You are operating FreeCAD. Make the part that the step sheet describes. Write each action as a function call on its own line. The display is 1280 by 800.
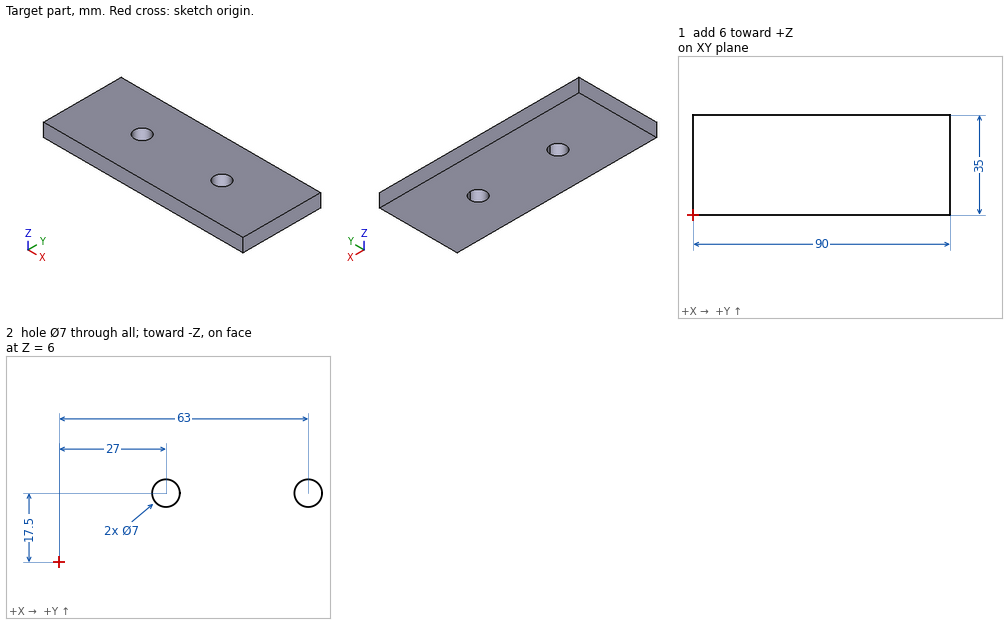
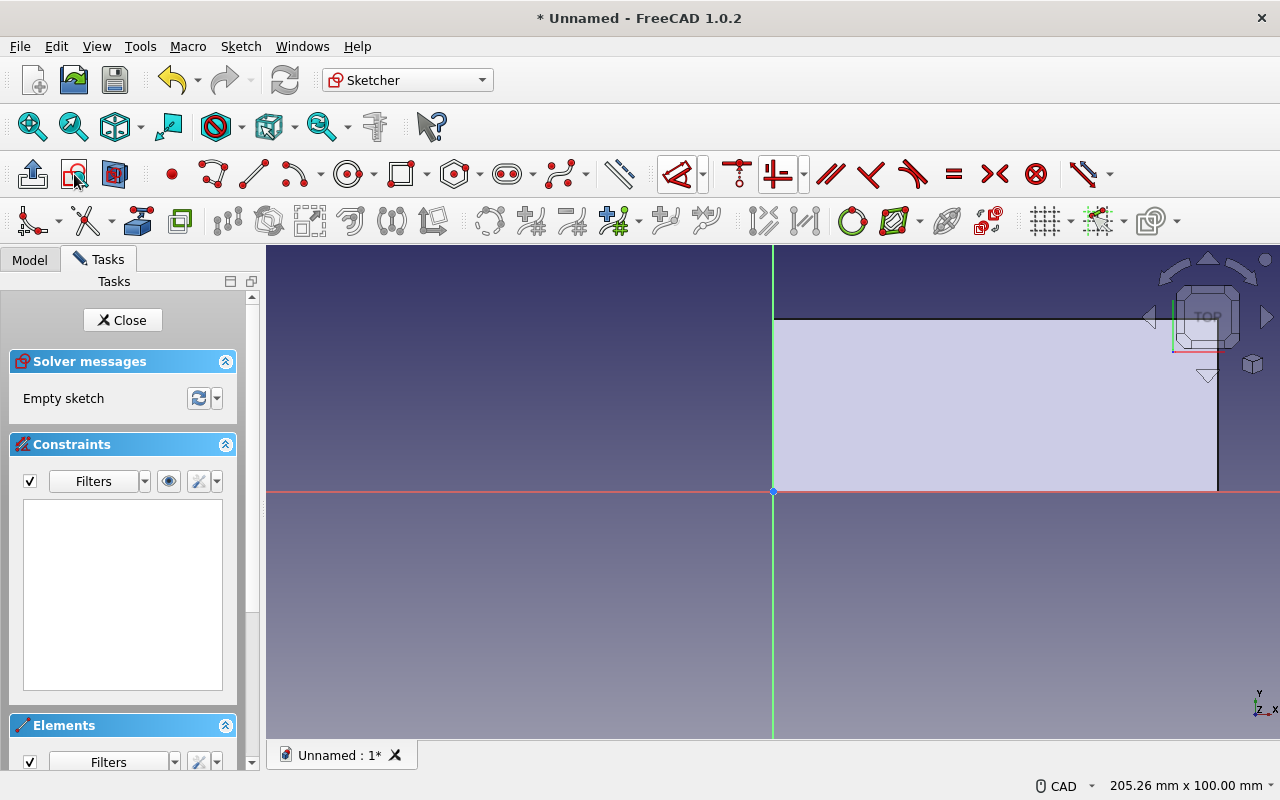
scroll(704, 492, down, 5)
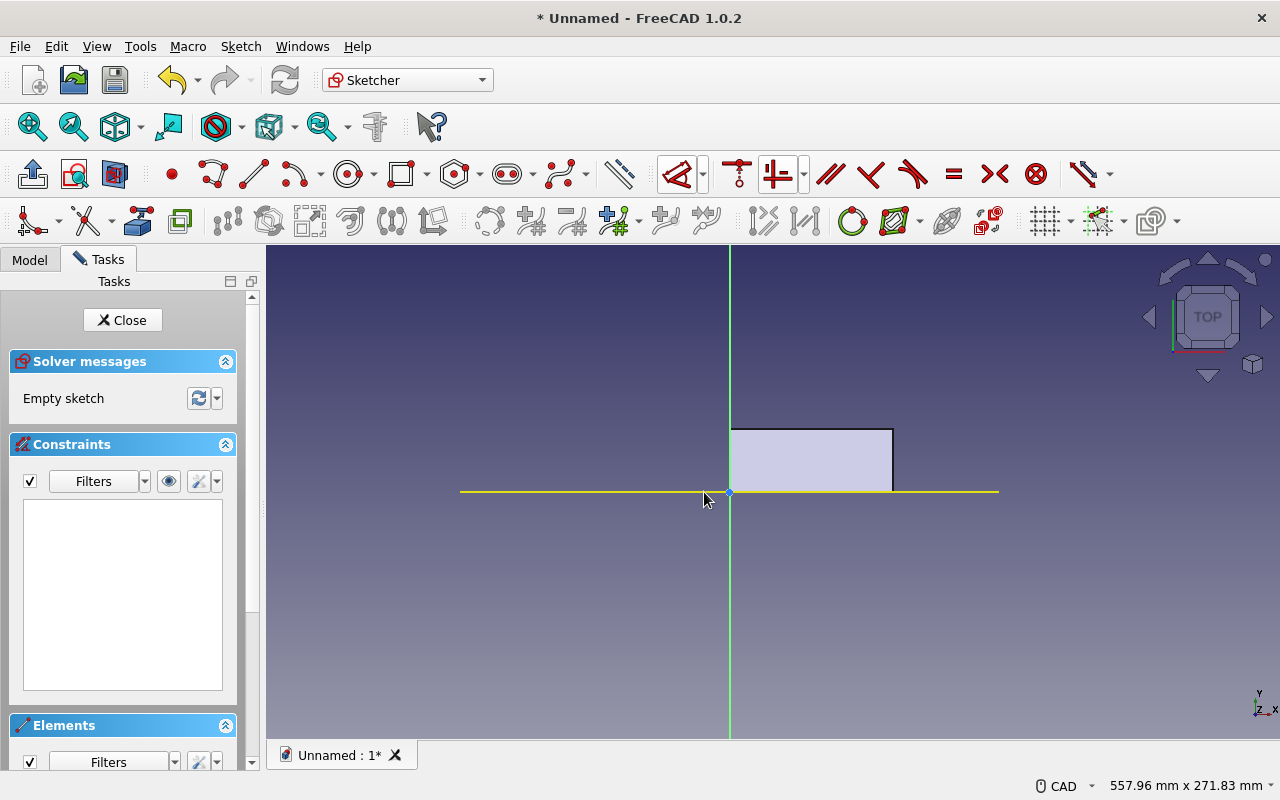
scroll(812, 468, up, 8)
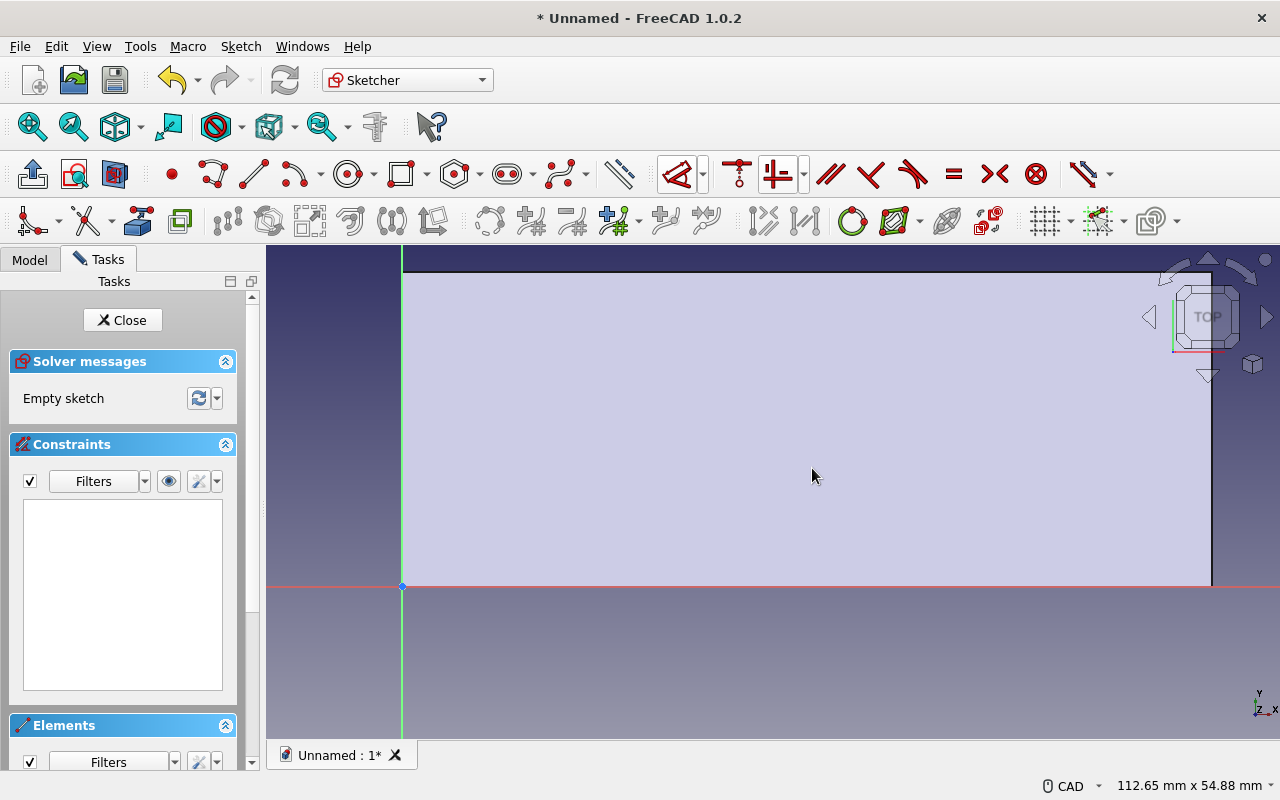
click(348, 174)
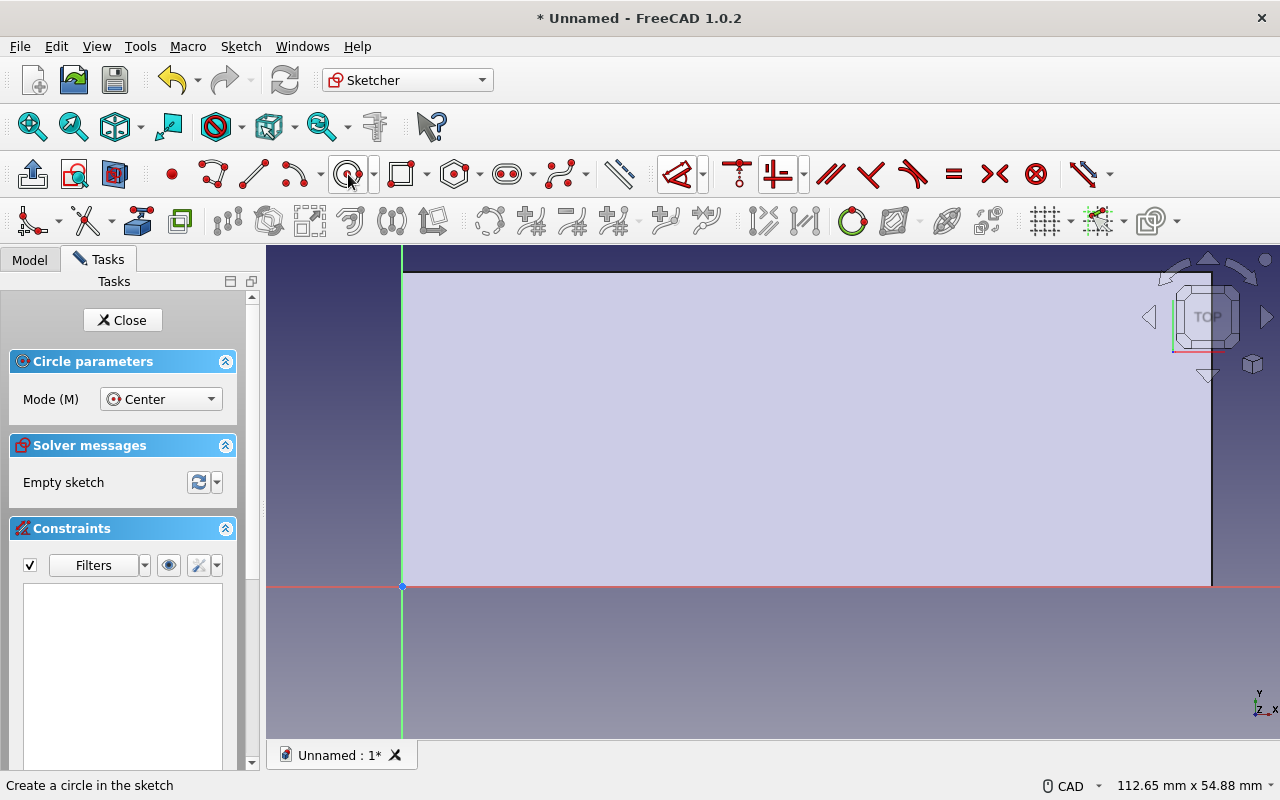
click(645, 429)
click(667, 407)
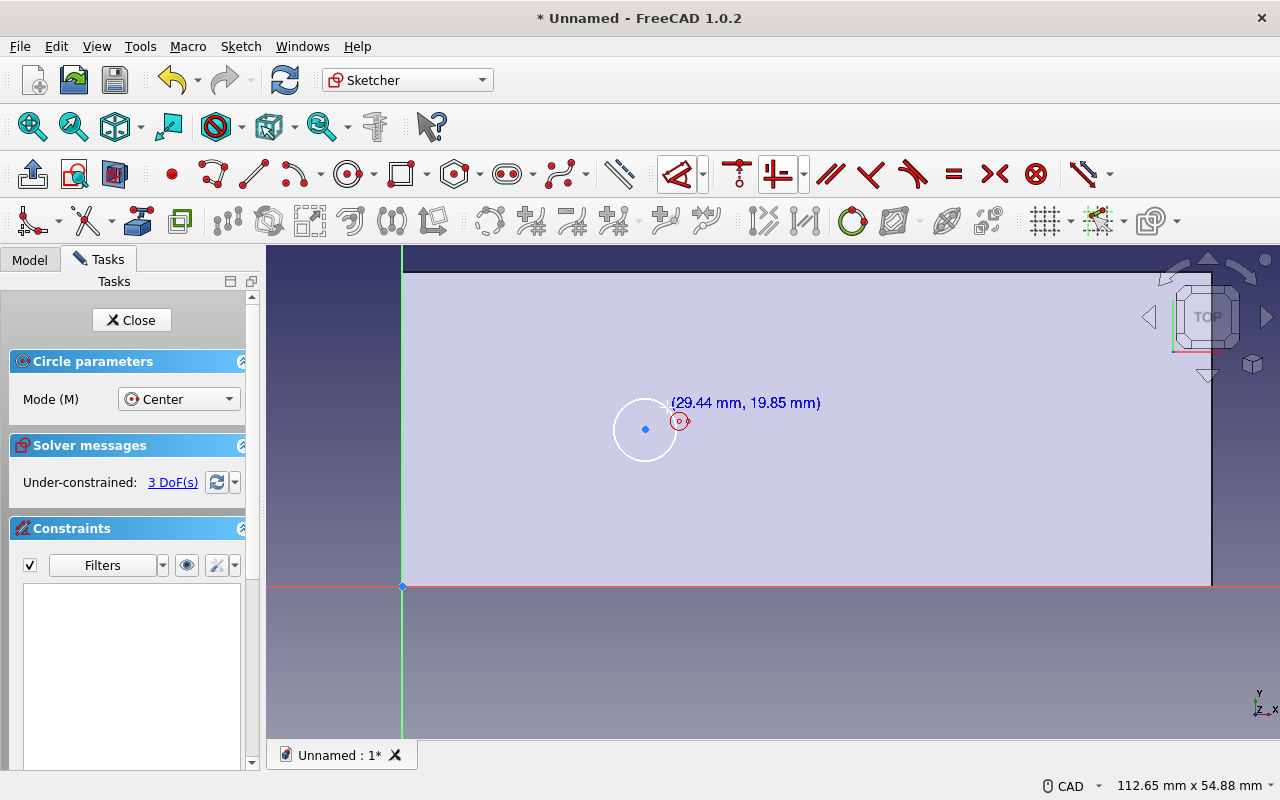
click(969, 429)
click(991, 407)
key(Escape)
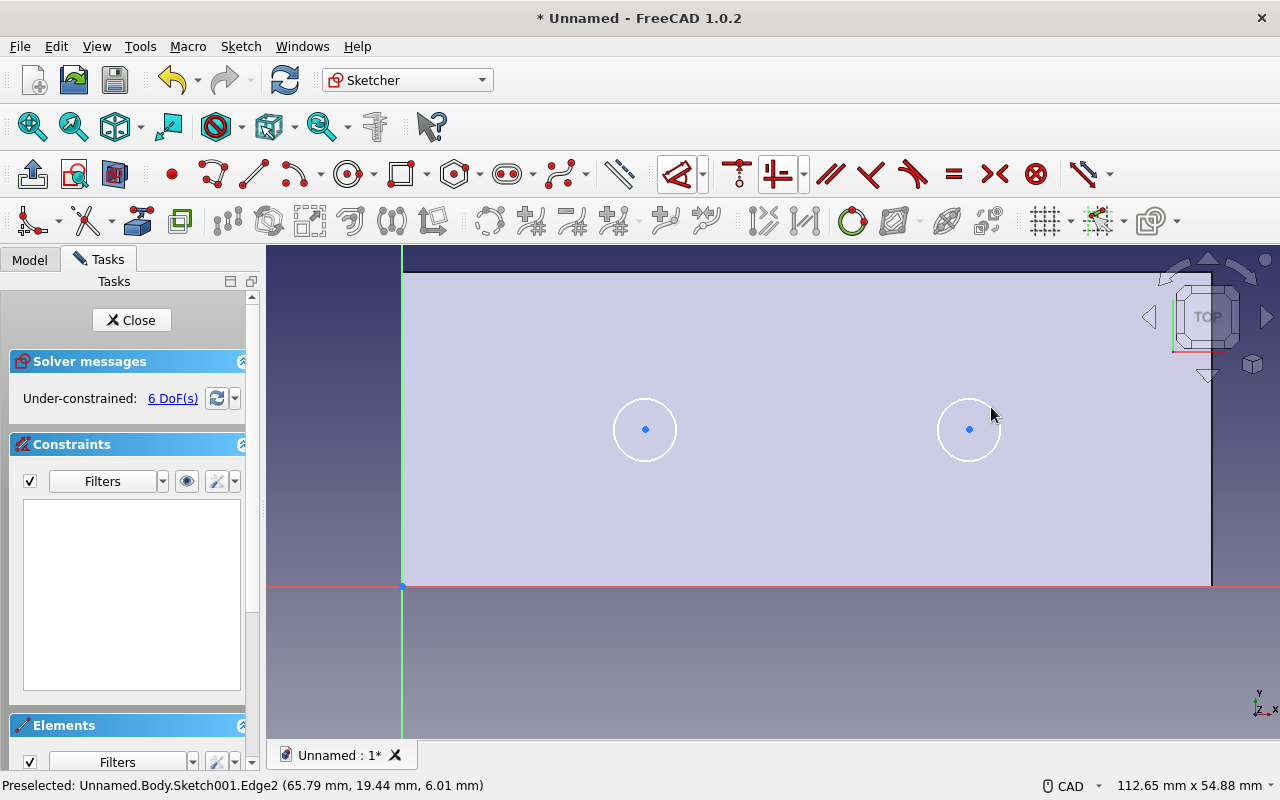
click(667, 408)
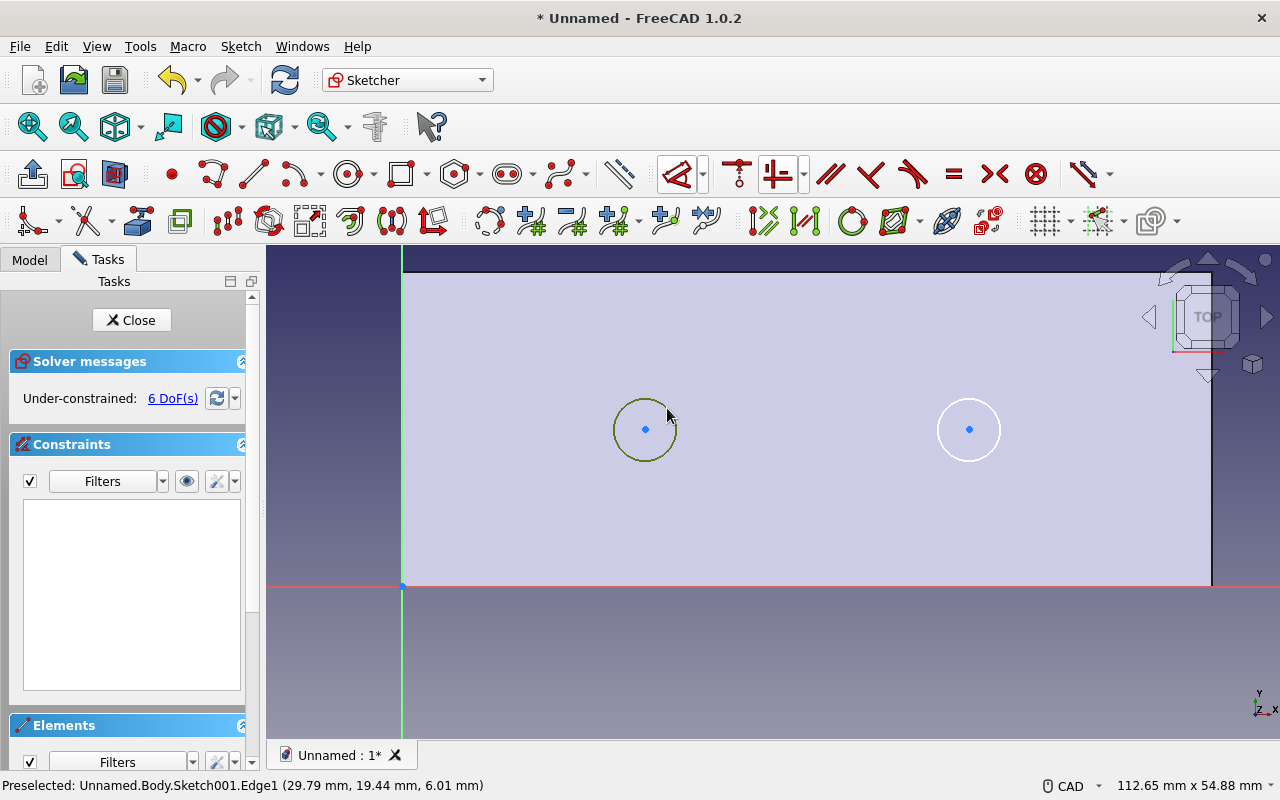
click(991, 408)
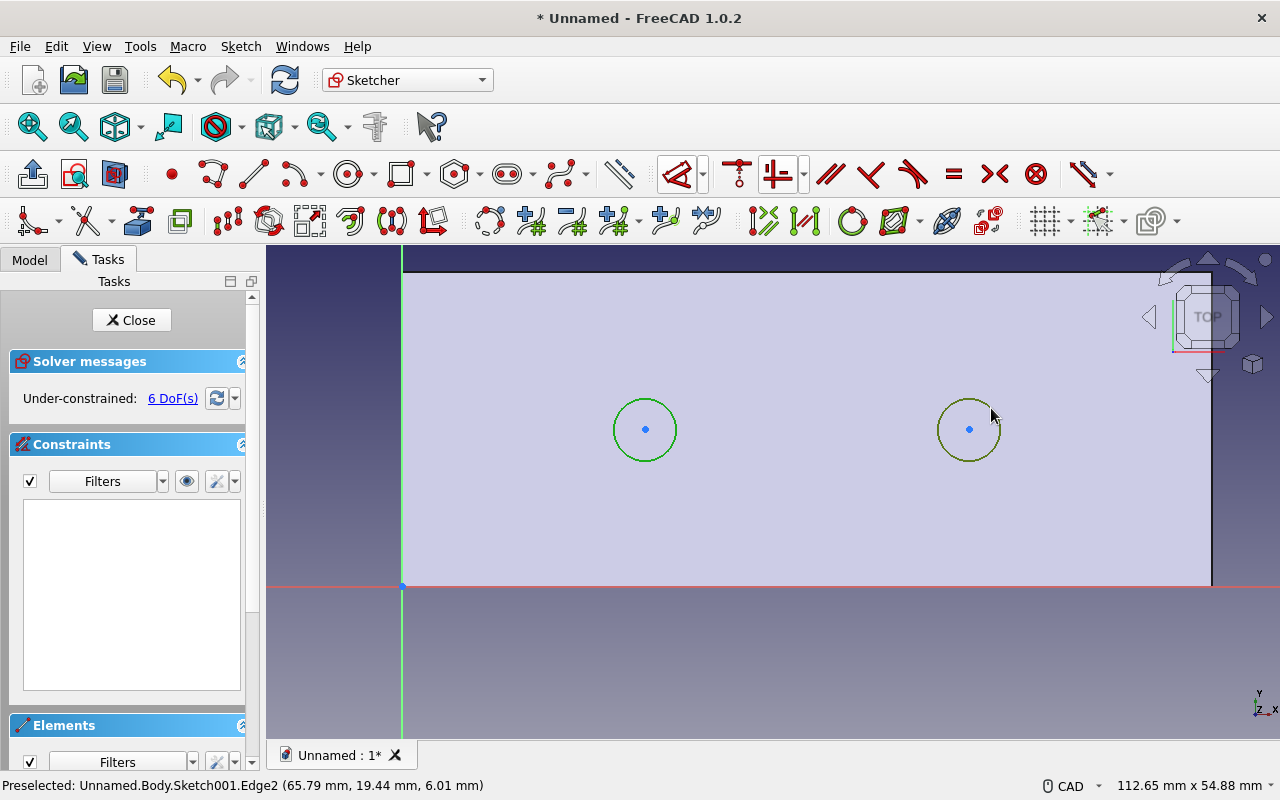
click(954, 174)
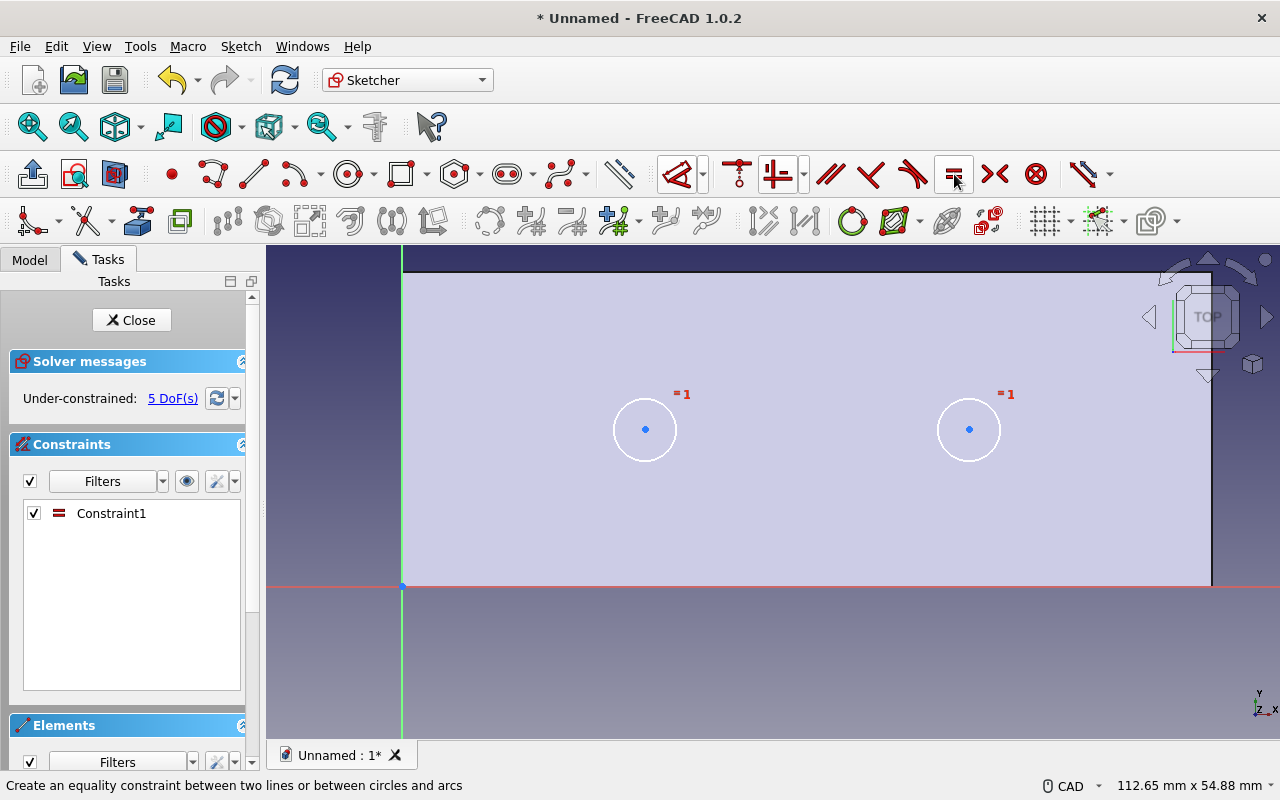
click(645, 430)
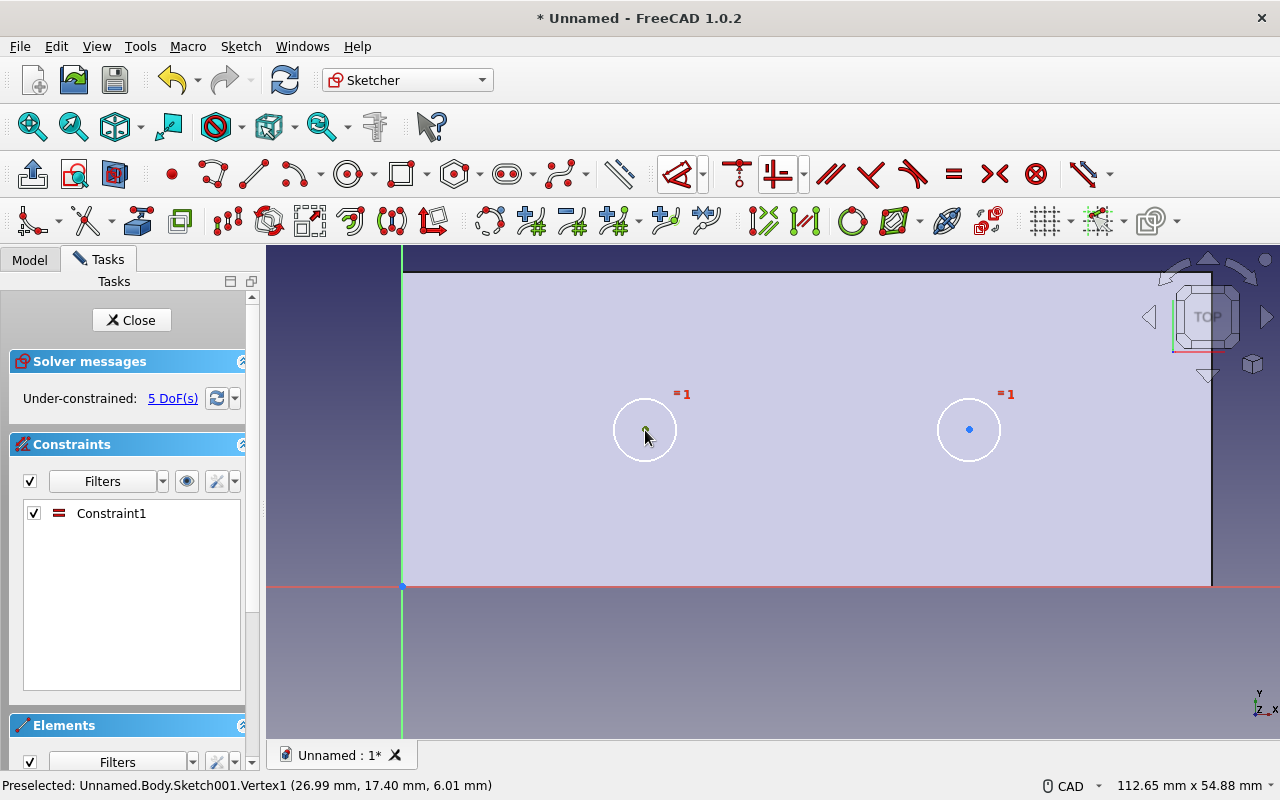
click(969, 430)